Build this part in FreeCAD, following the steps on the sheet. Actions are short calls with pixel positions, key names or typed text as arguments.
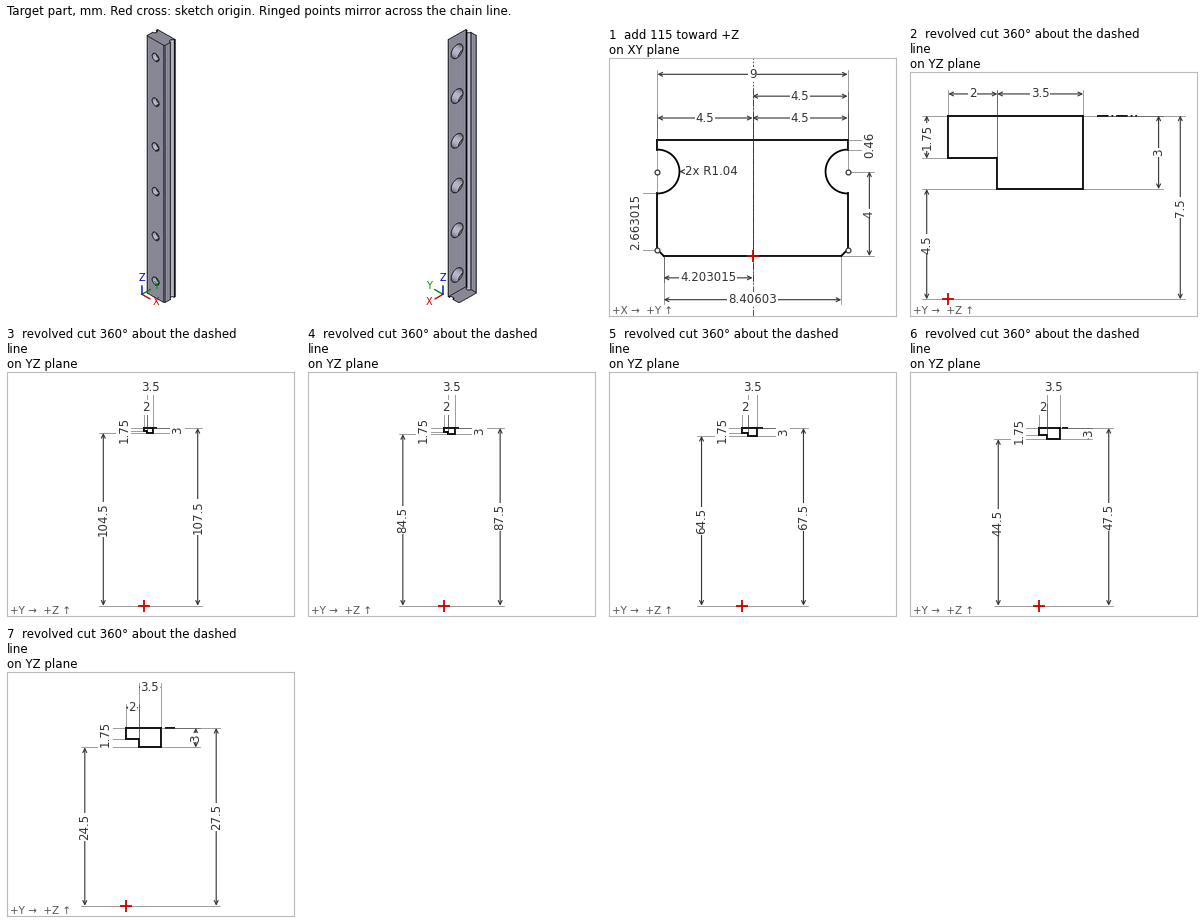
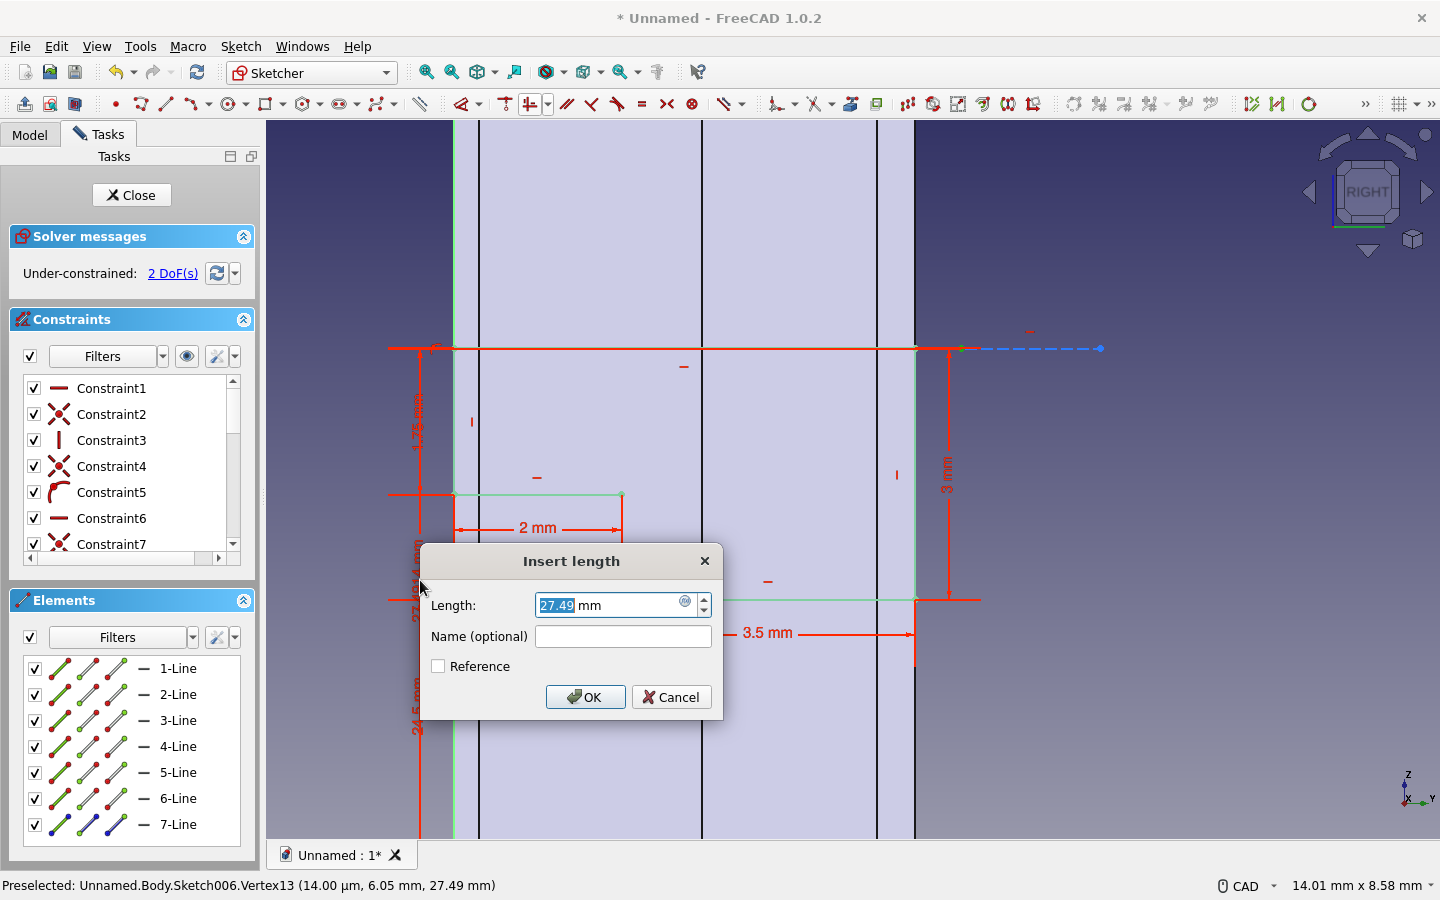
text(27.5)
key(Return)
key(Escape)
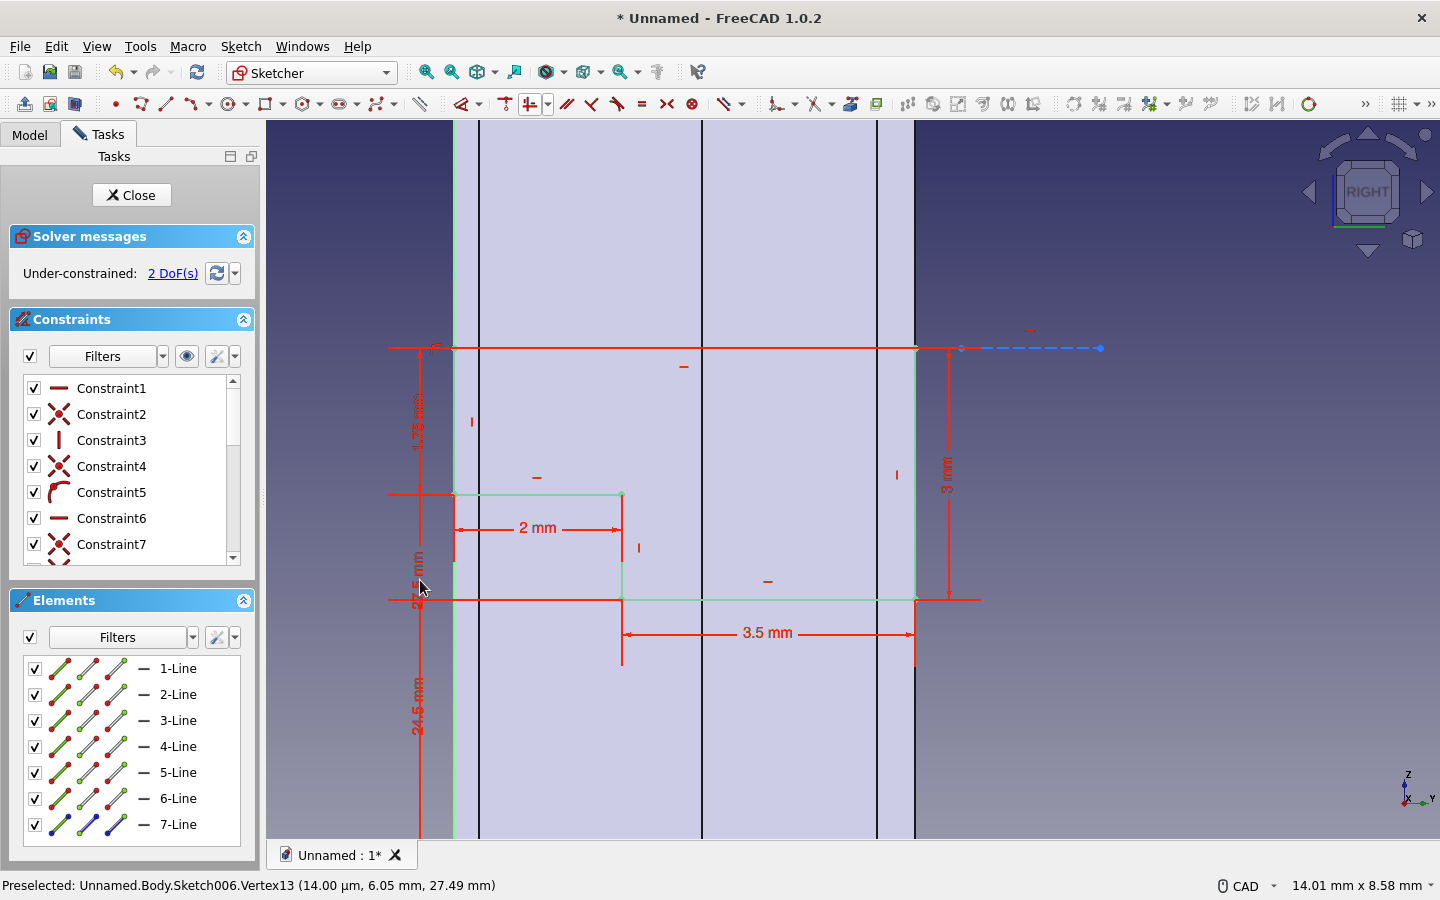
click(132, 195)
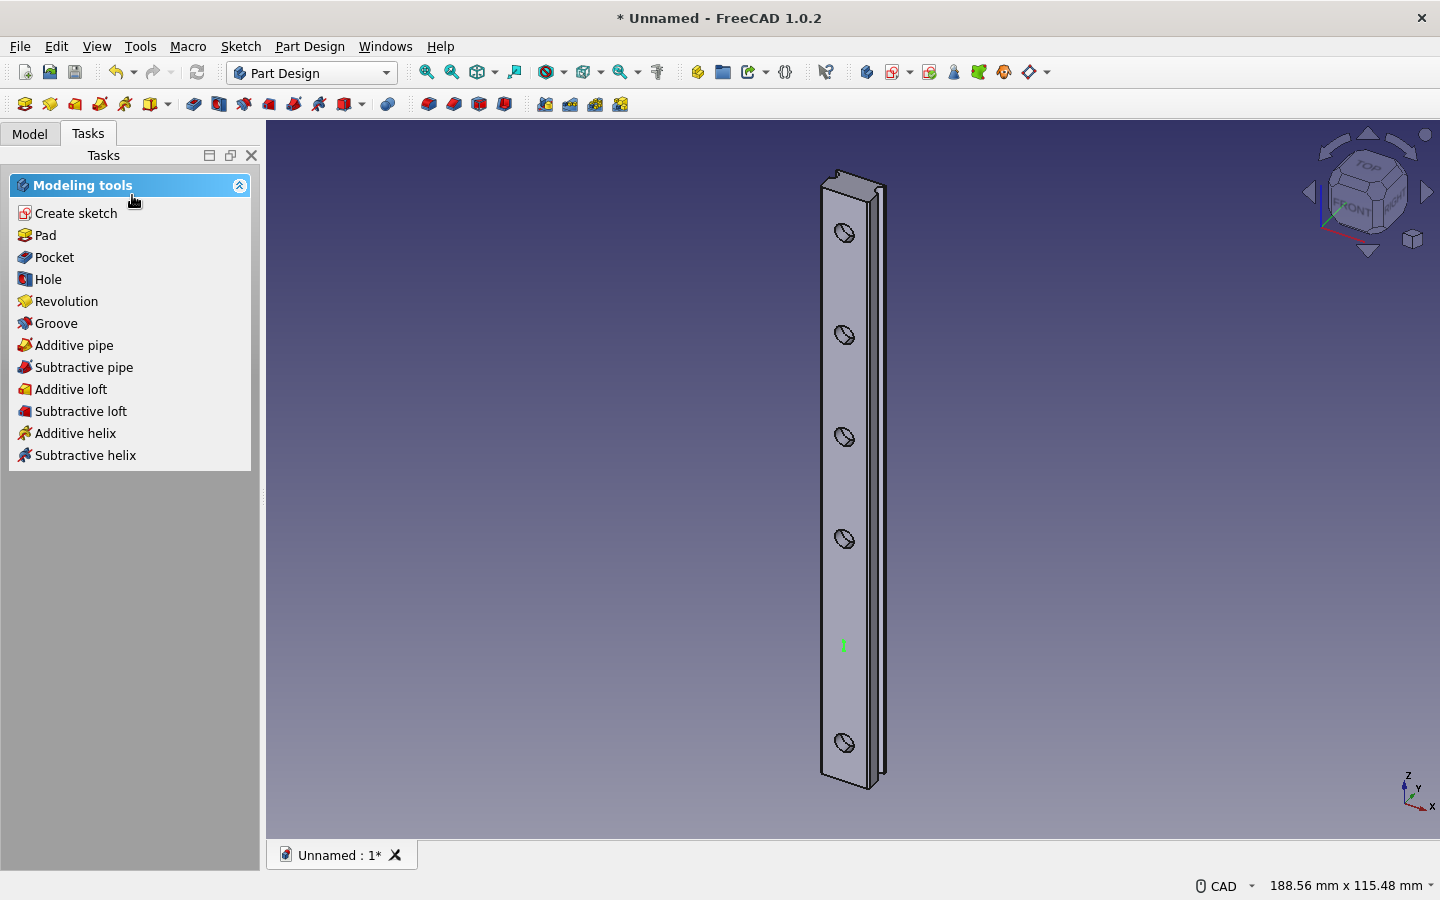
click(244, 104)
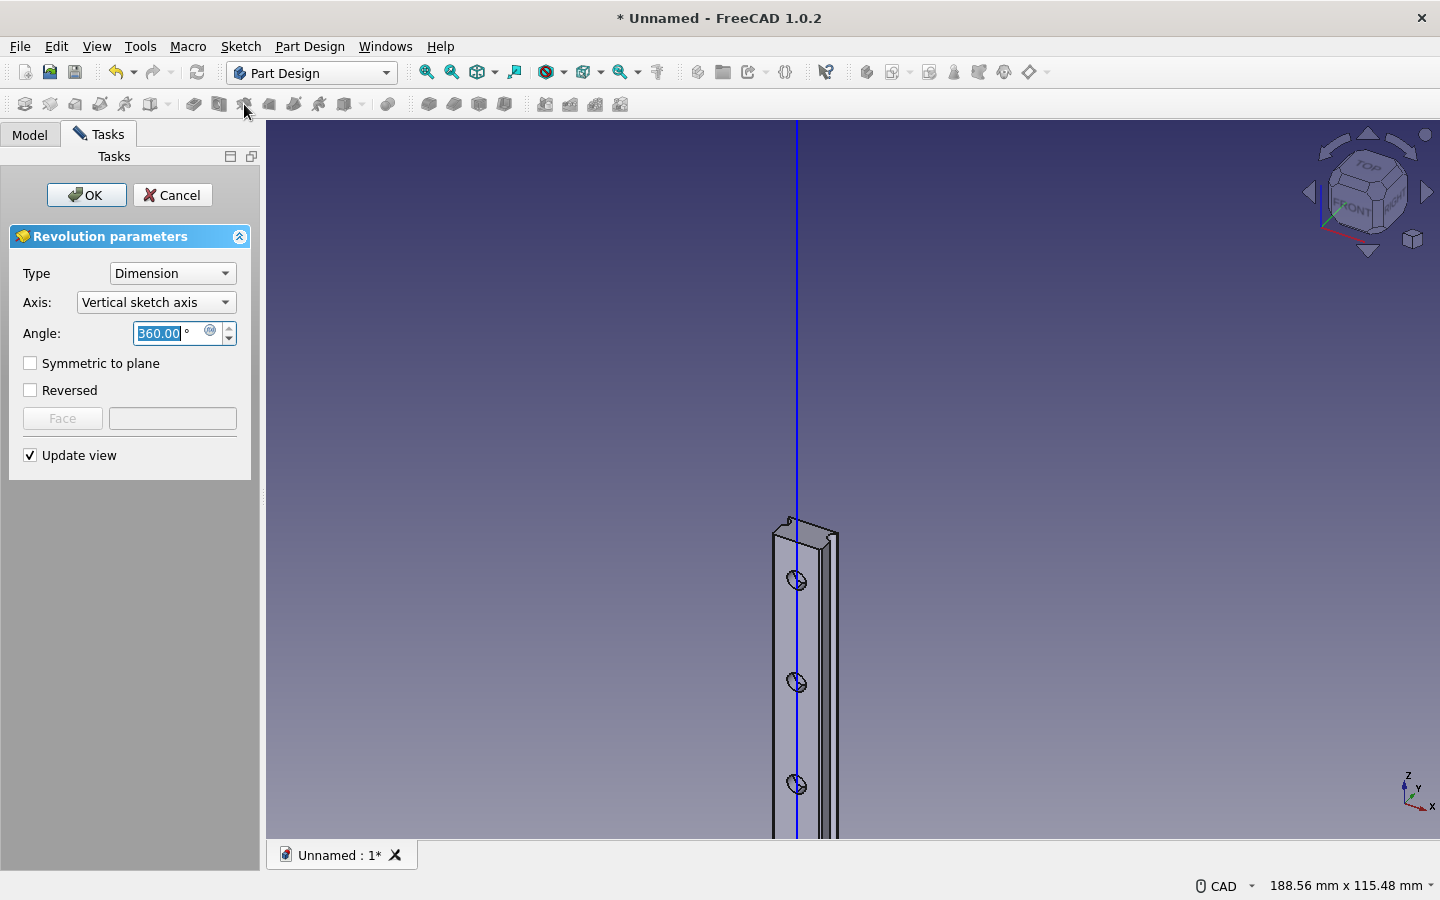
click(157, 302)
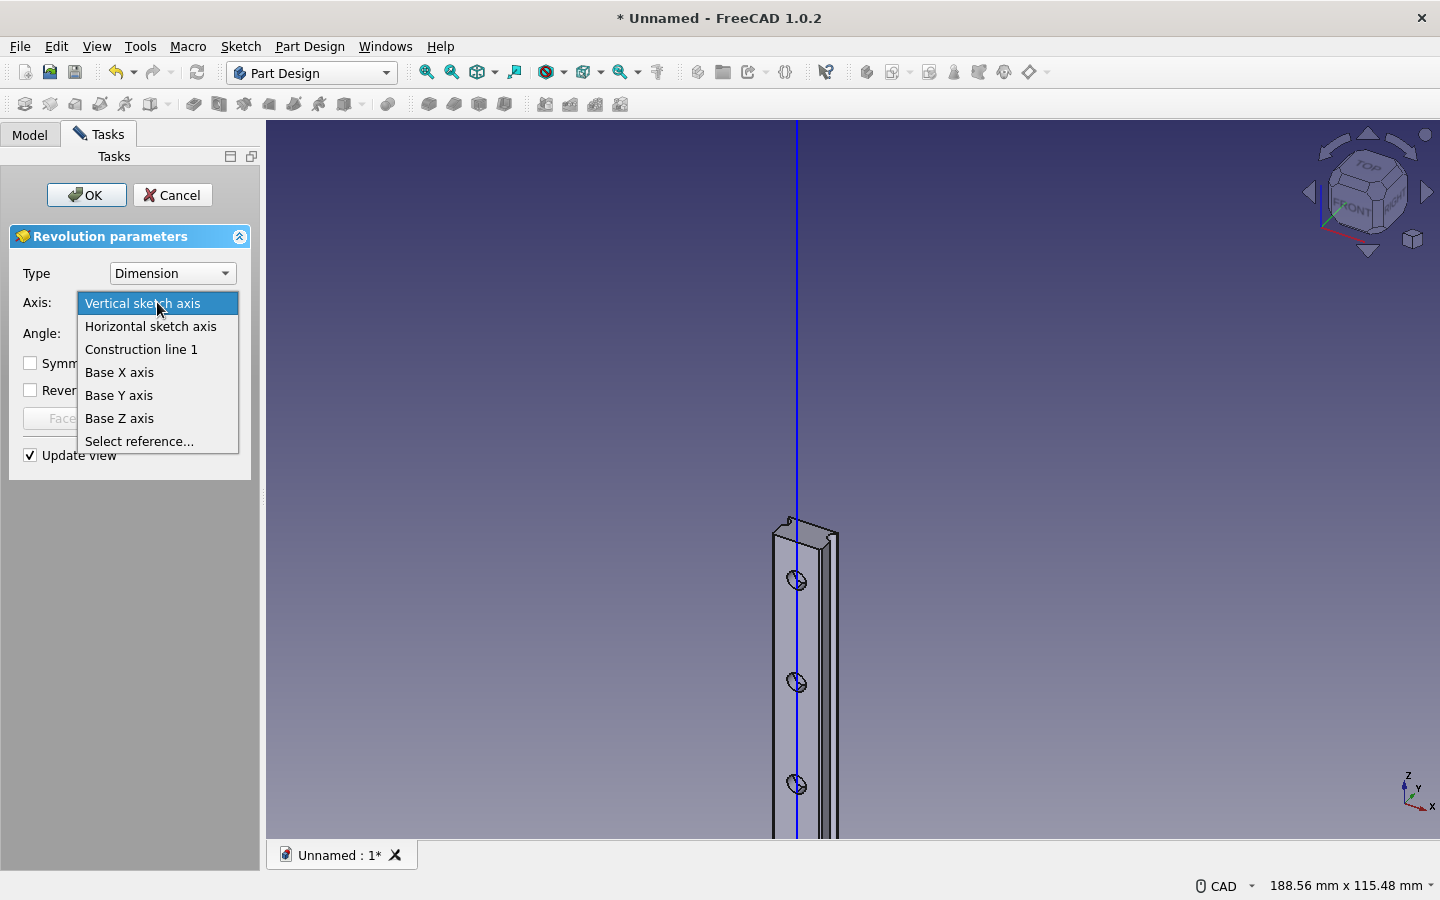
click(156, 350)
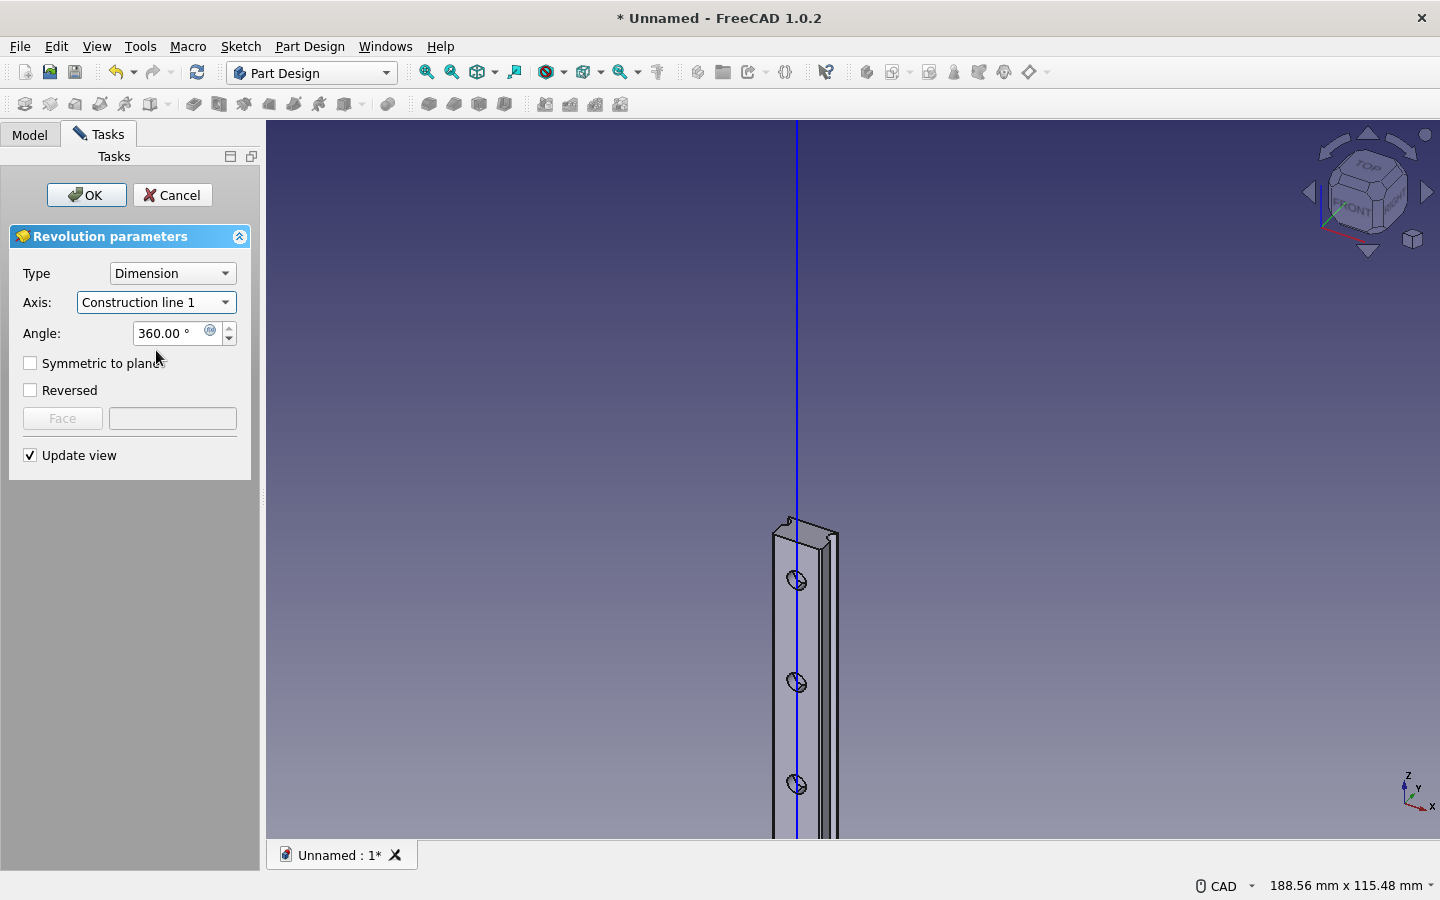
click(87, 195)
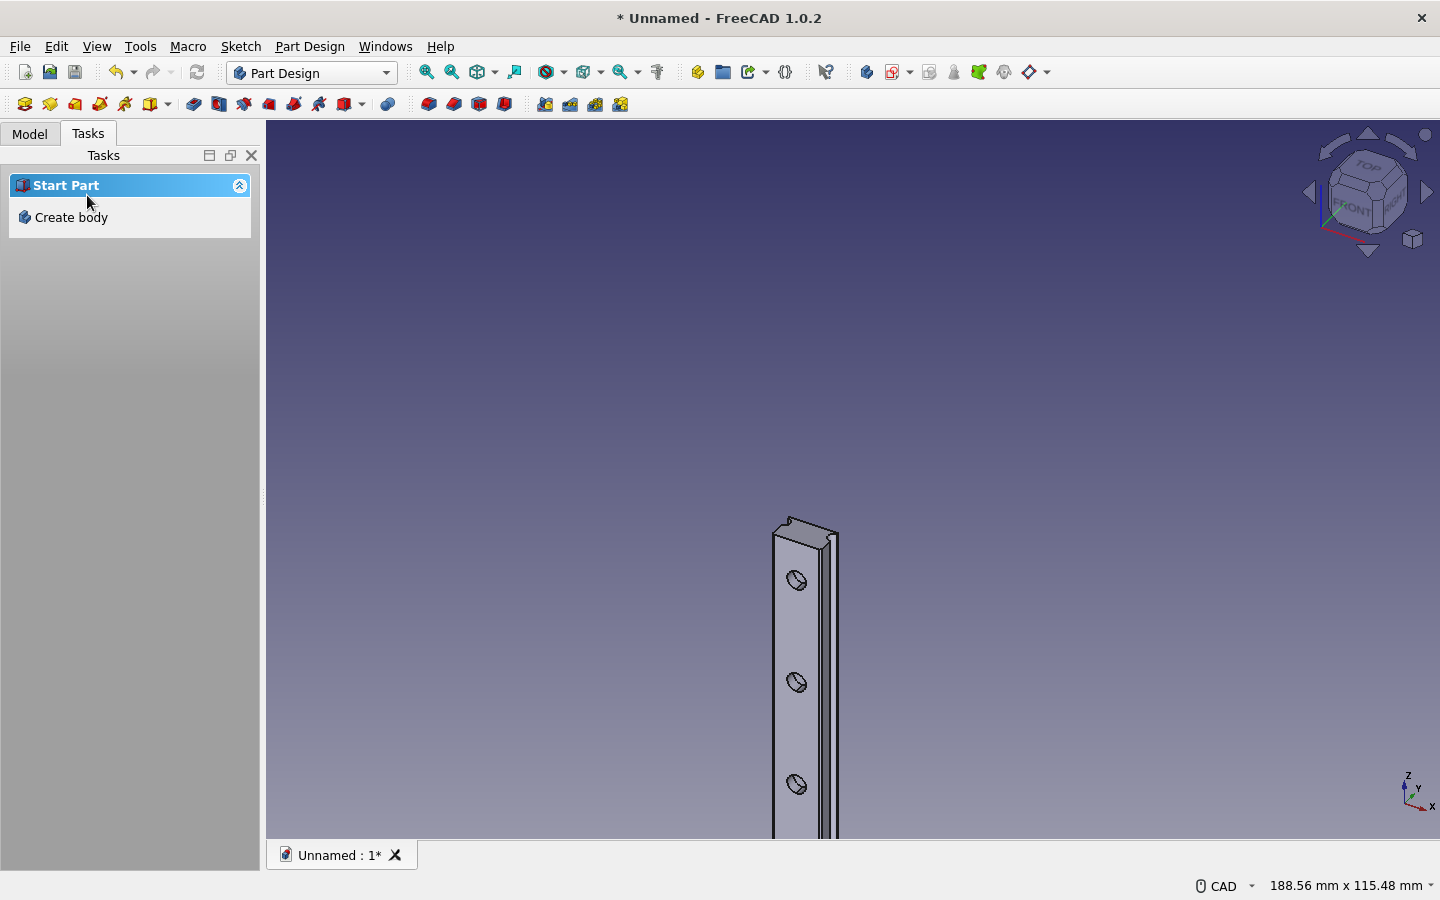
key(0)